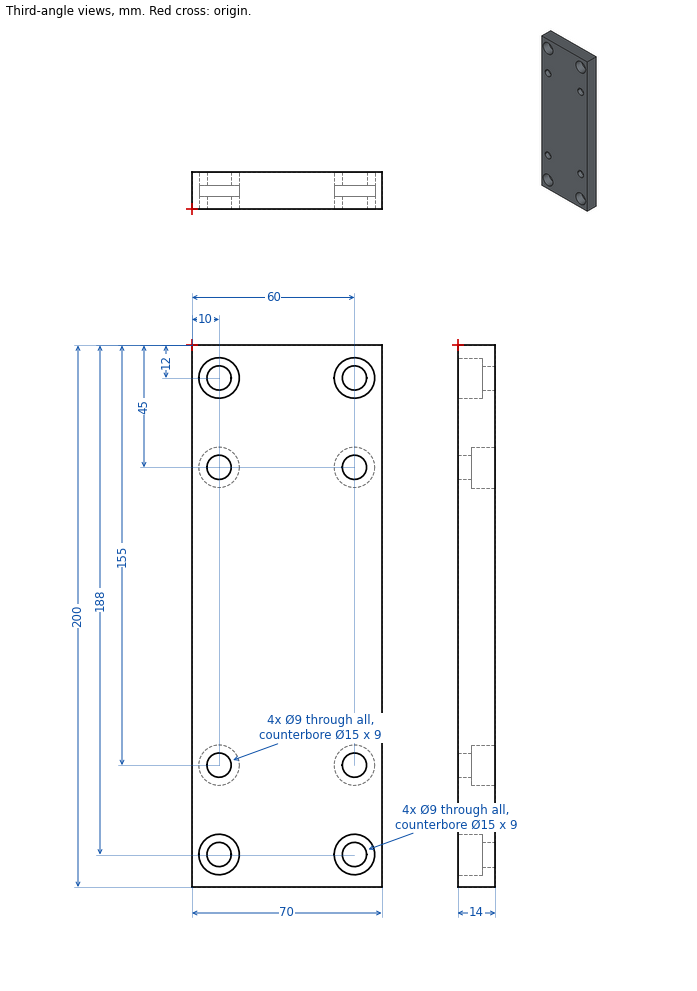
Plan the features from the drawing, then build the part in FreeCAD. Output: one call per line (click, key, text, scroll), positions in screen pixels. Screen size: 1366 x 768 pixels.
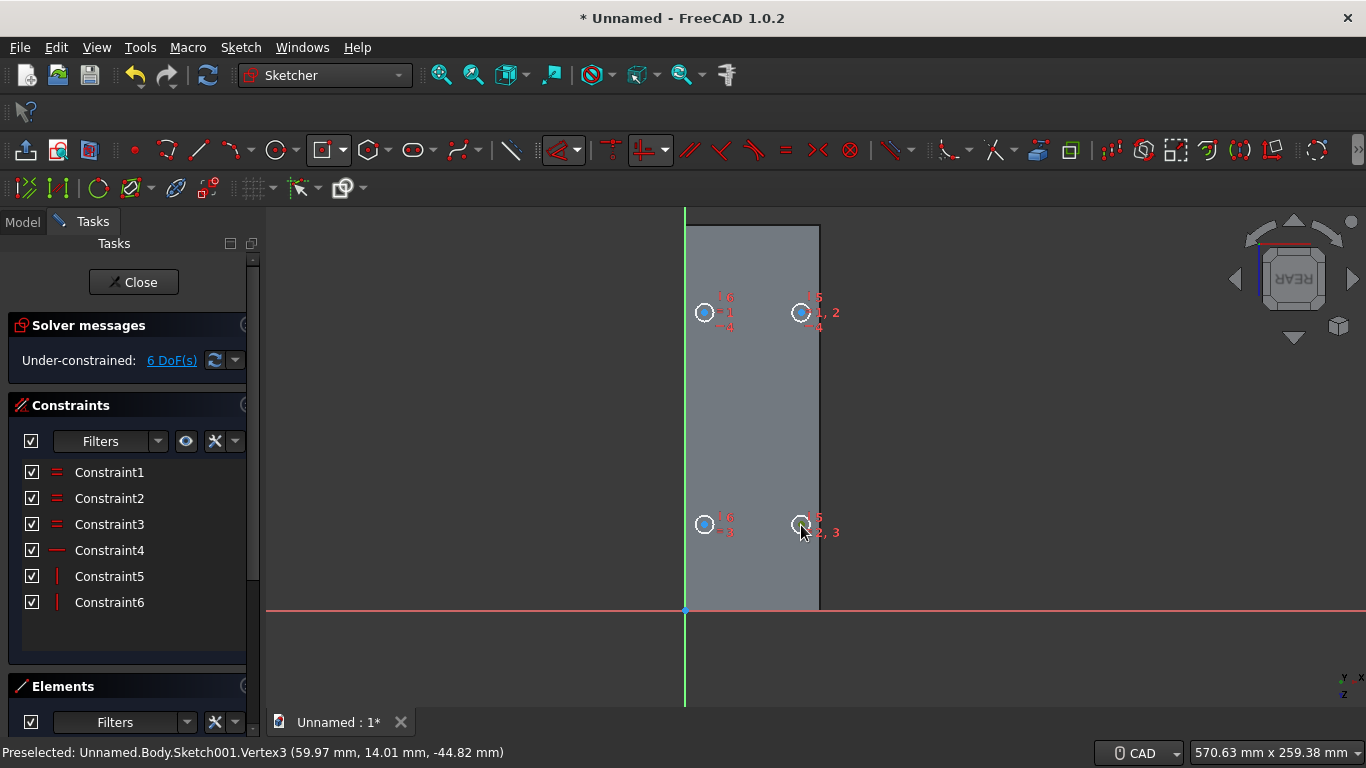
click(705, 525)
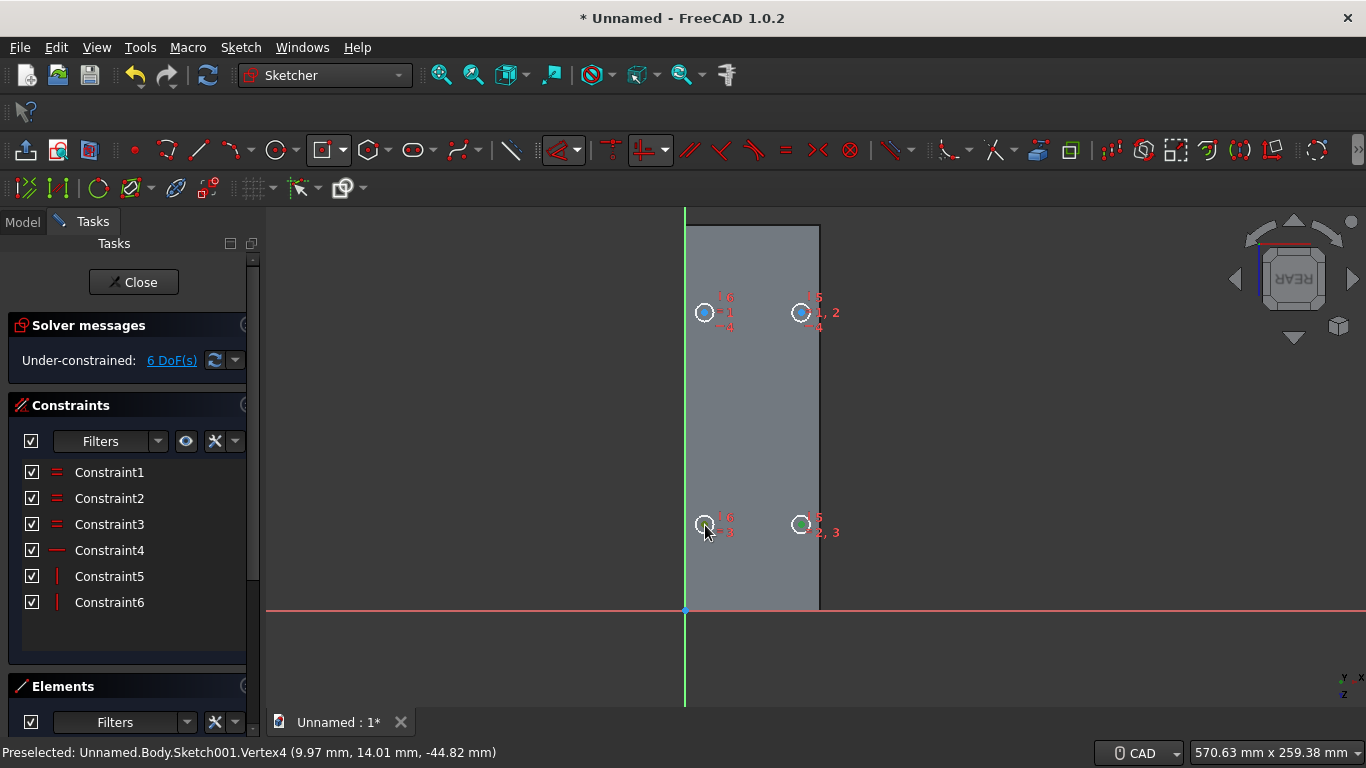
key(h)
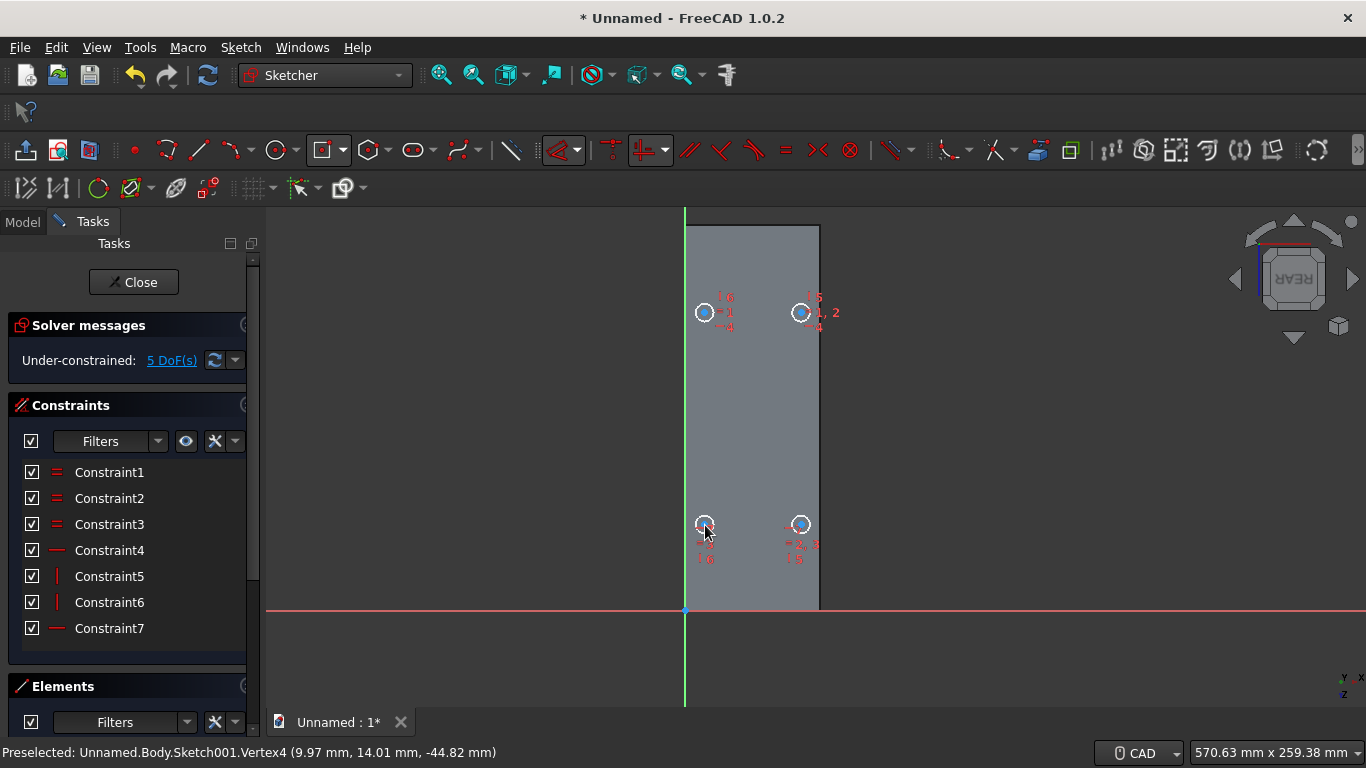
key(d)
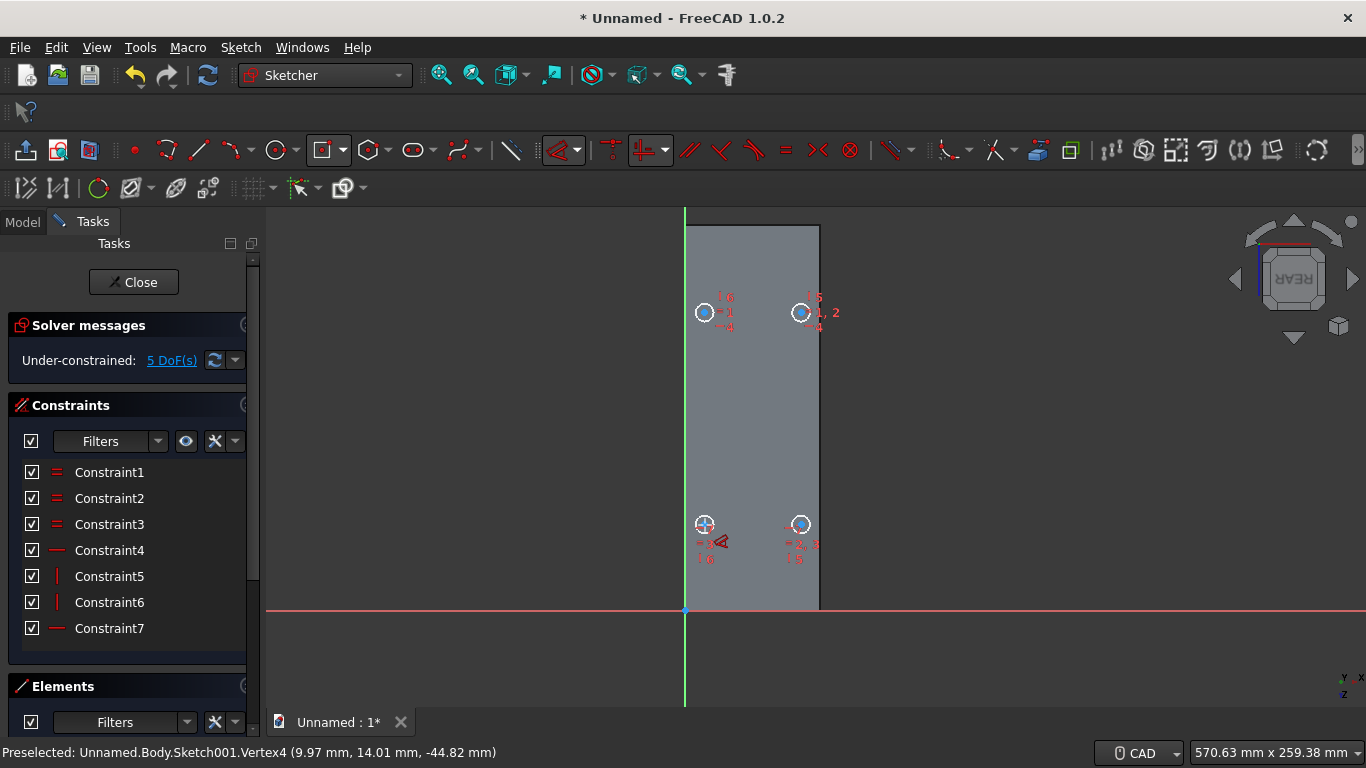
scroll(711, 306, up, 5)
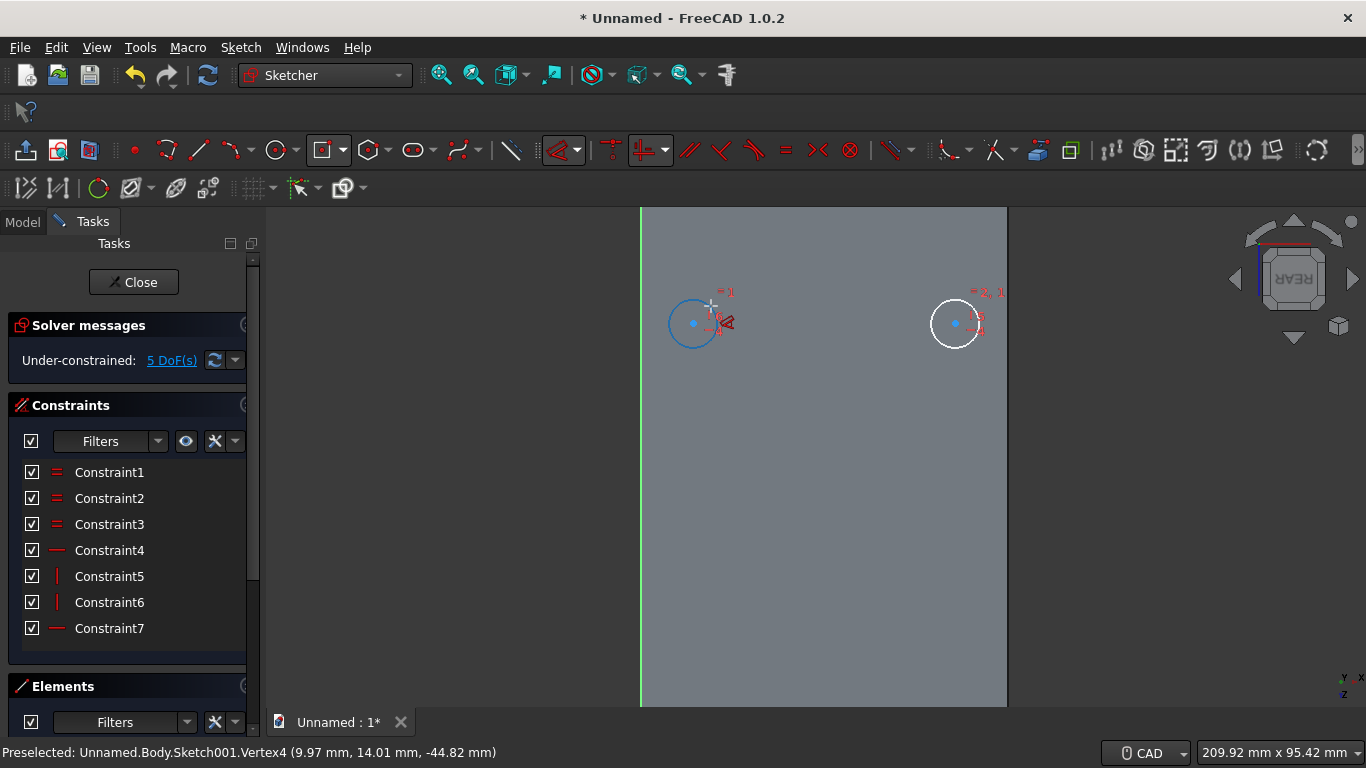
click(710, 307)
click(733, 284)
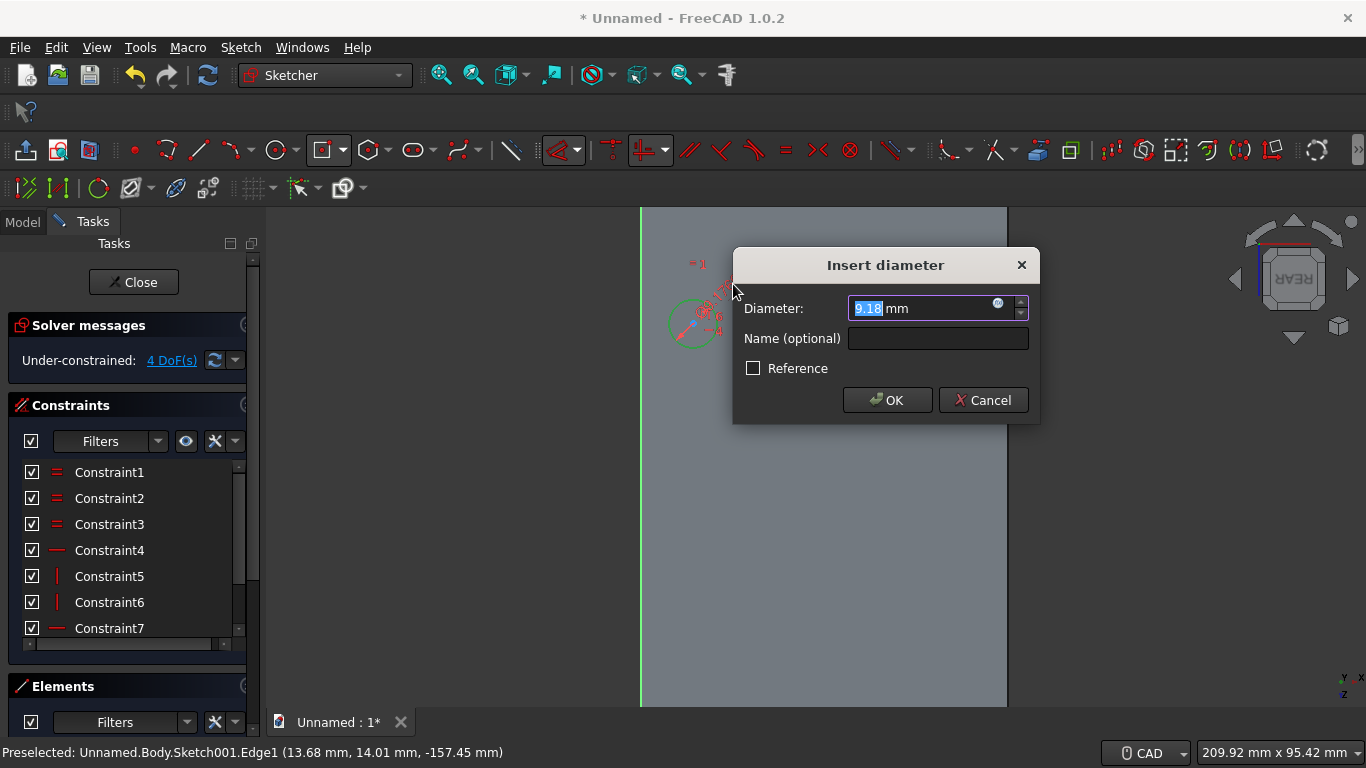
text(9)
key(Return)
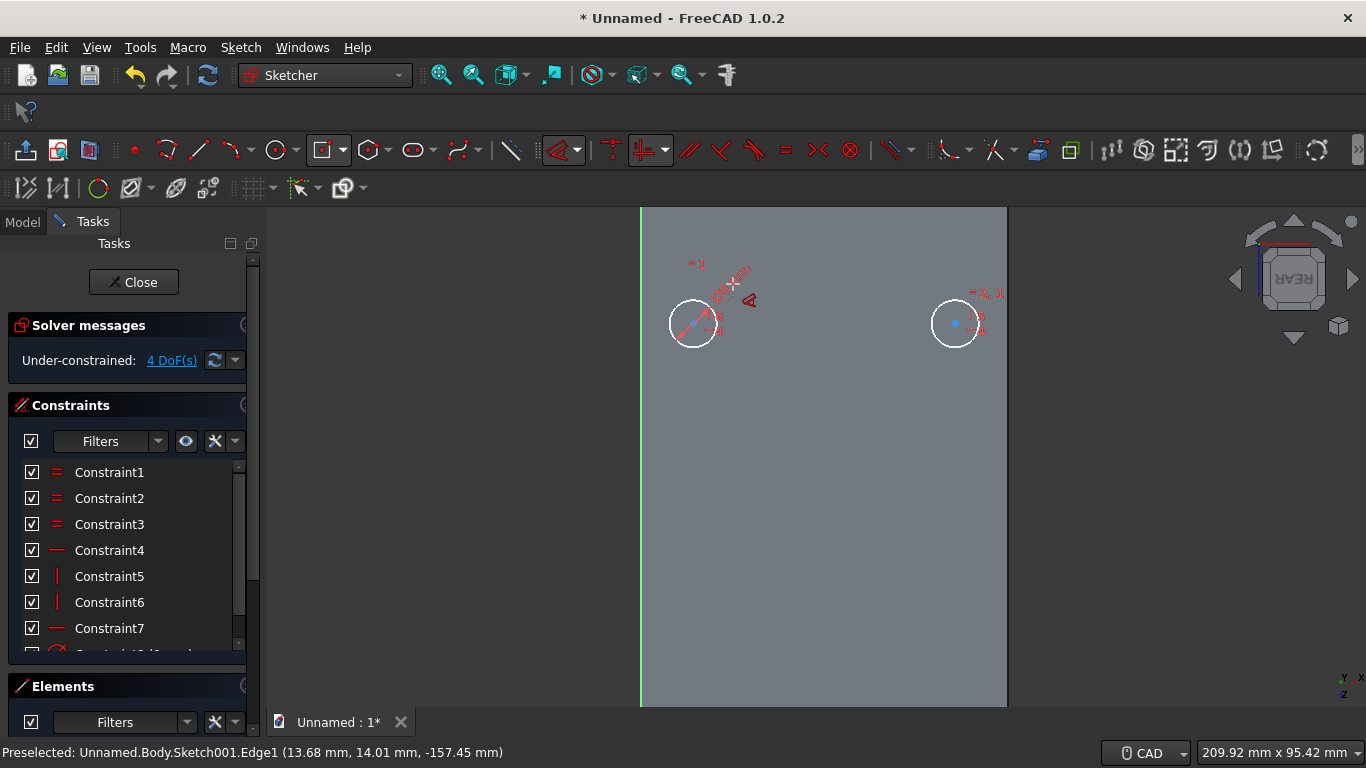
click(693, 324)
click(655, 290)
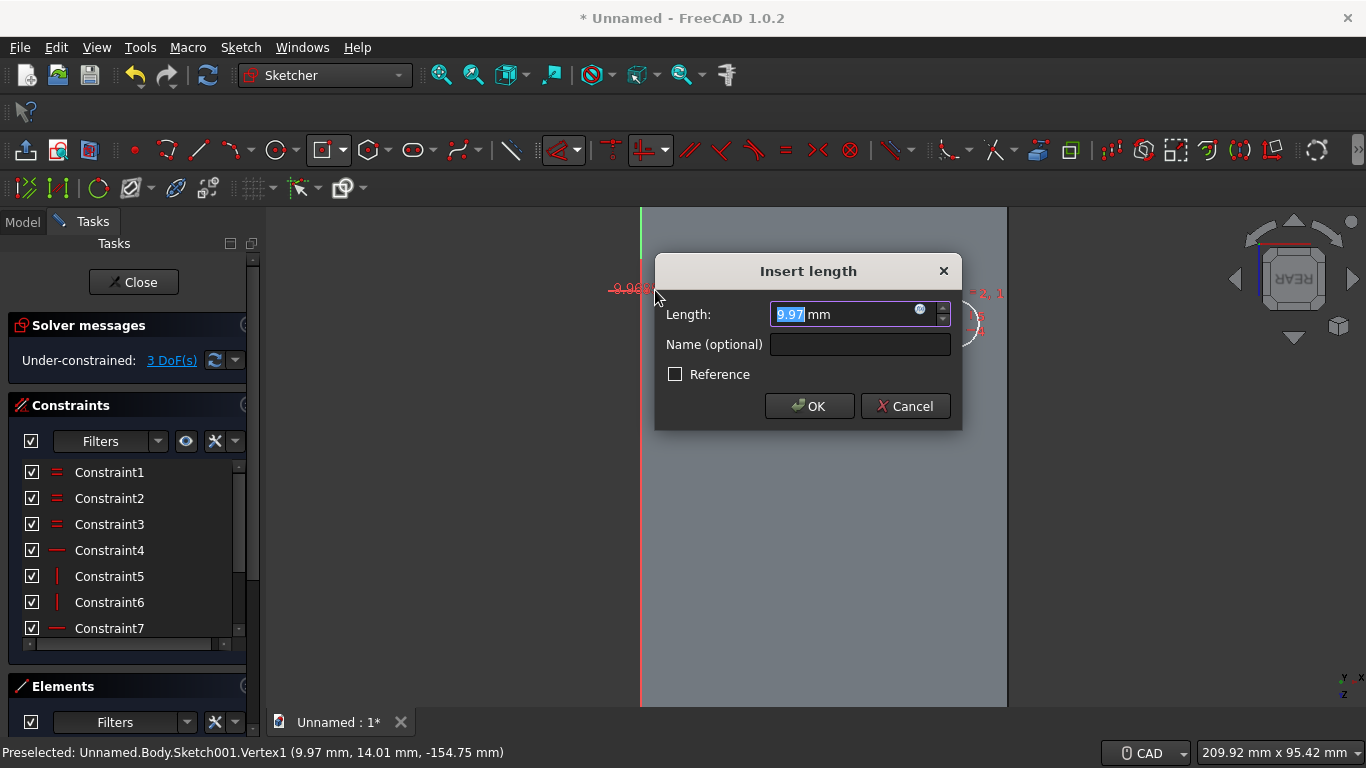
text(10)
key(Return)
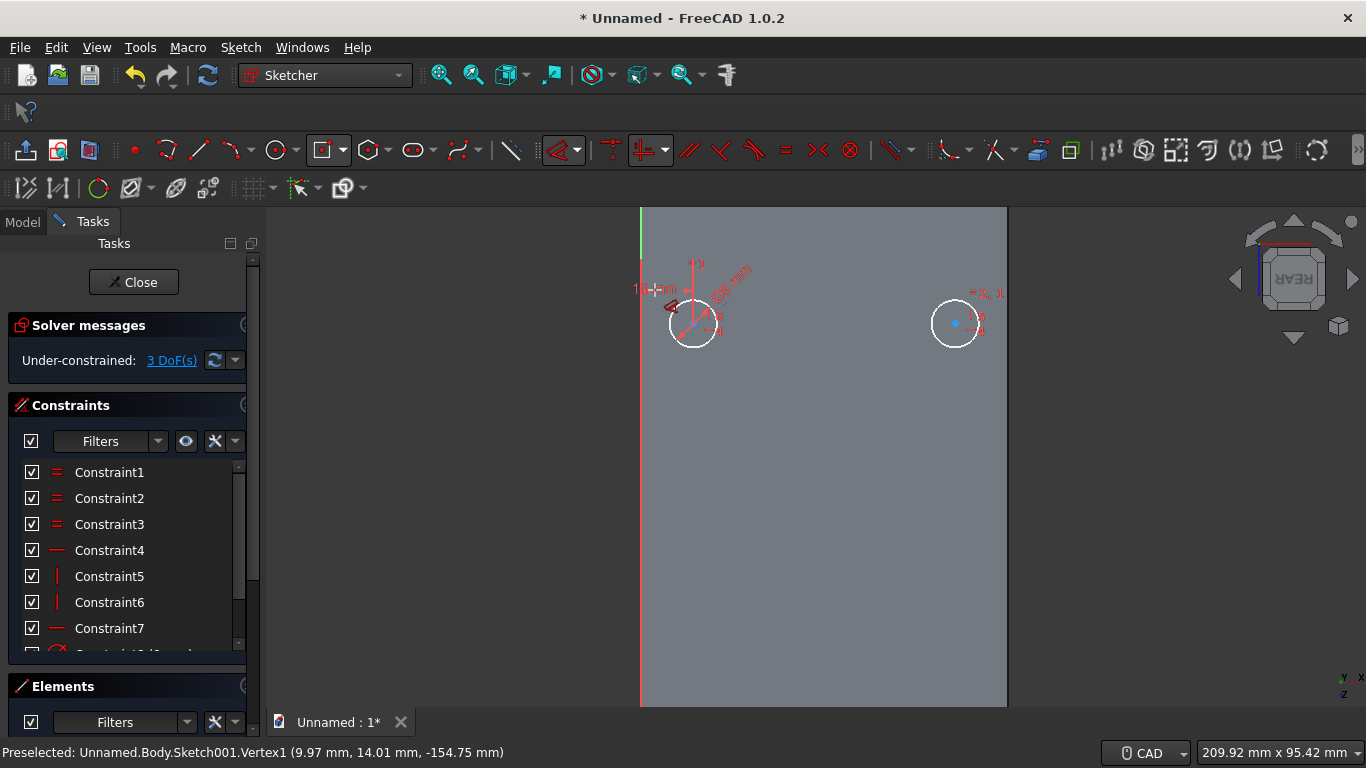
click(955, 324)
click(870, 290)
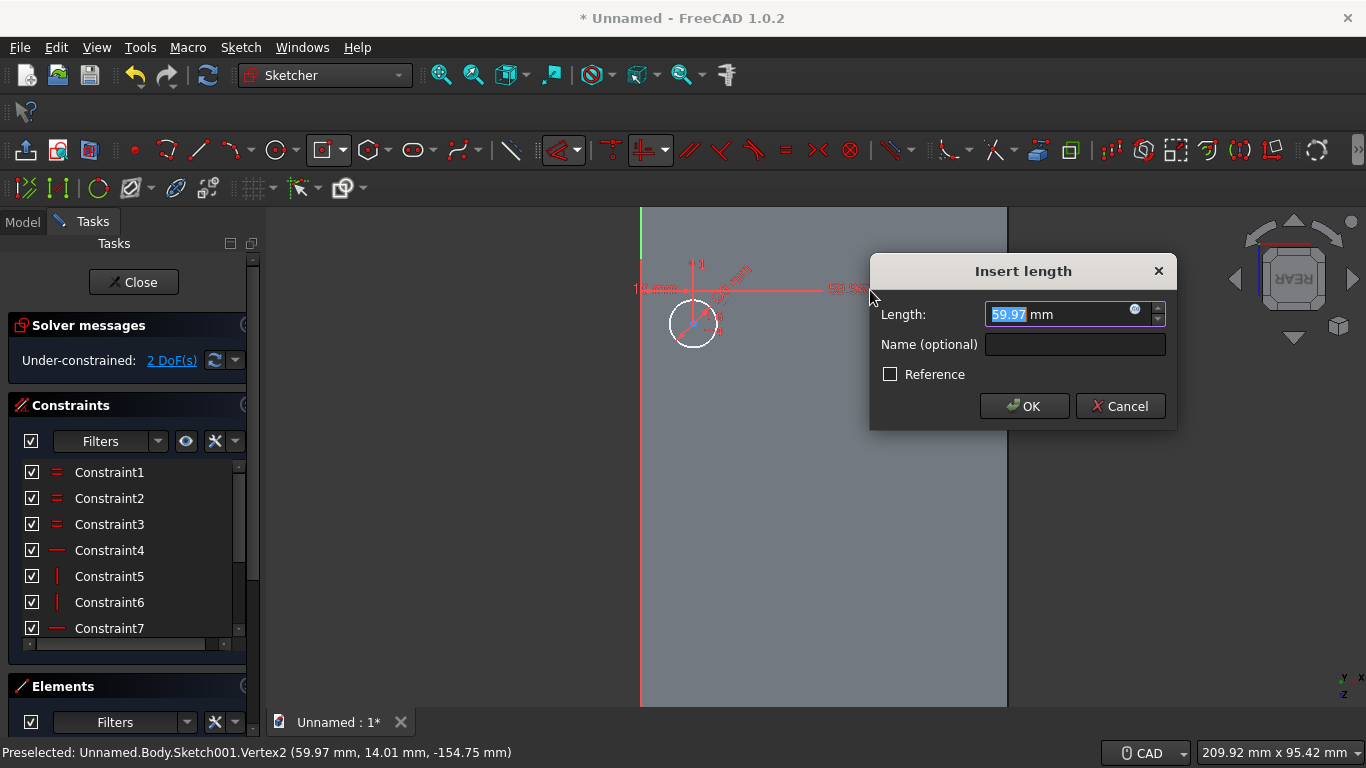
text(60)
key(Return)